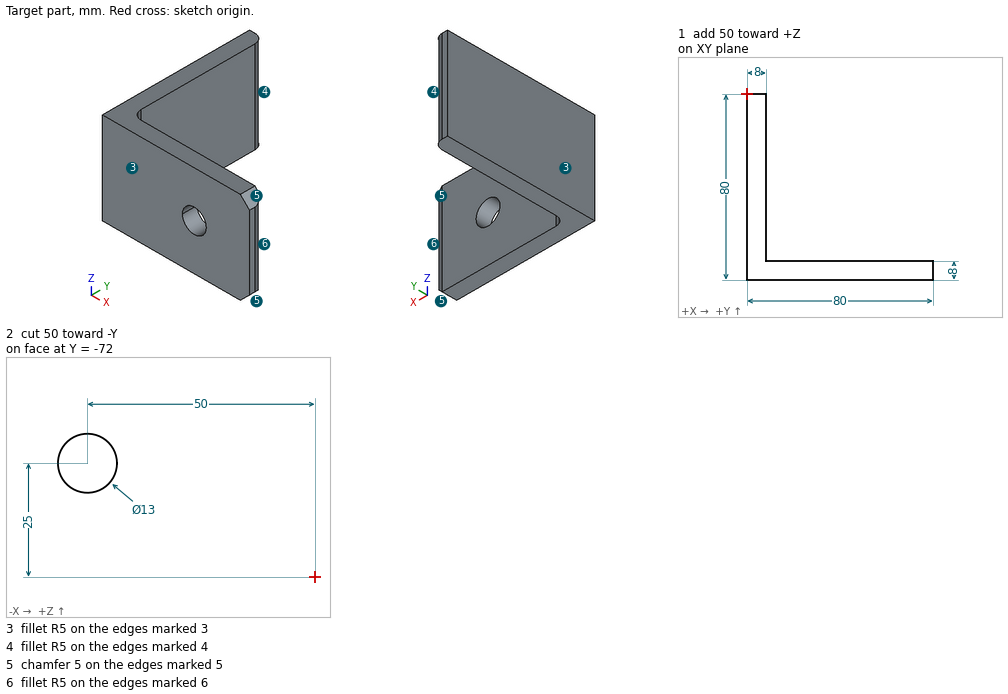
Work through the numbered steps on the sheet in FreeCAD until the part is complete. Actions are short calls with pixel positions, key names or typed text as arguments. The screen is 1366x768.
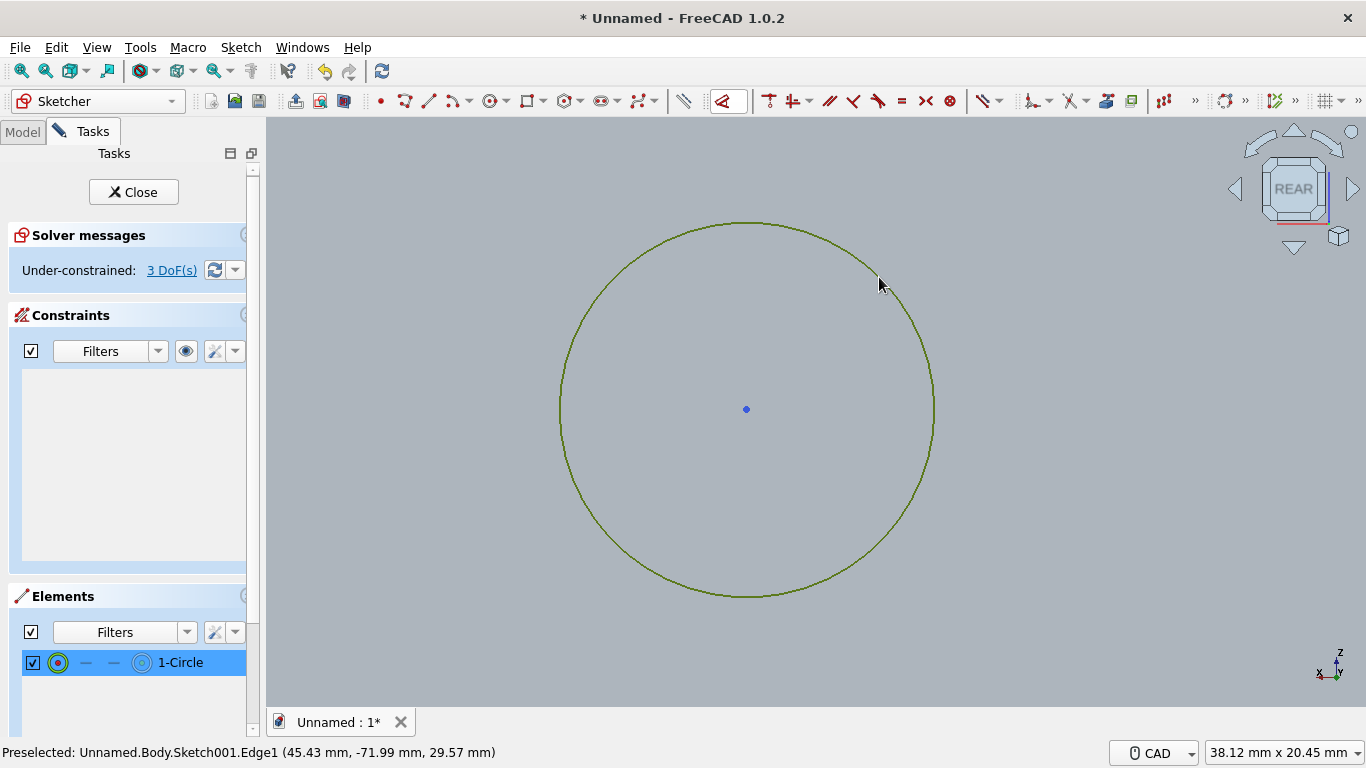
key(k)
key(o)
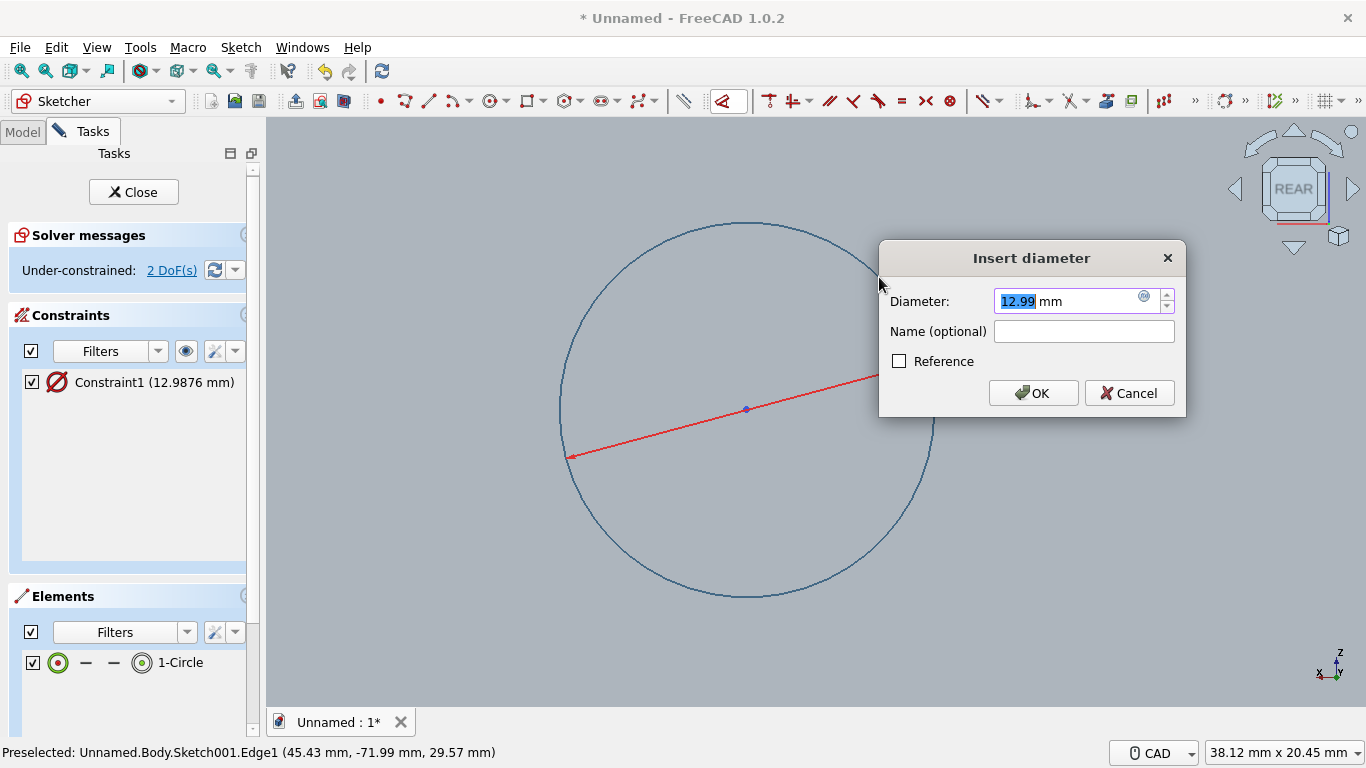
text(13)
key(Return)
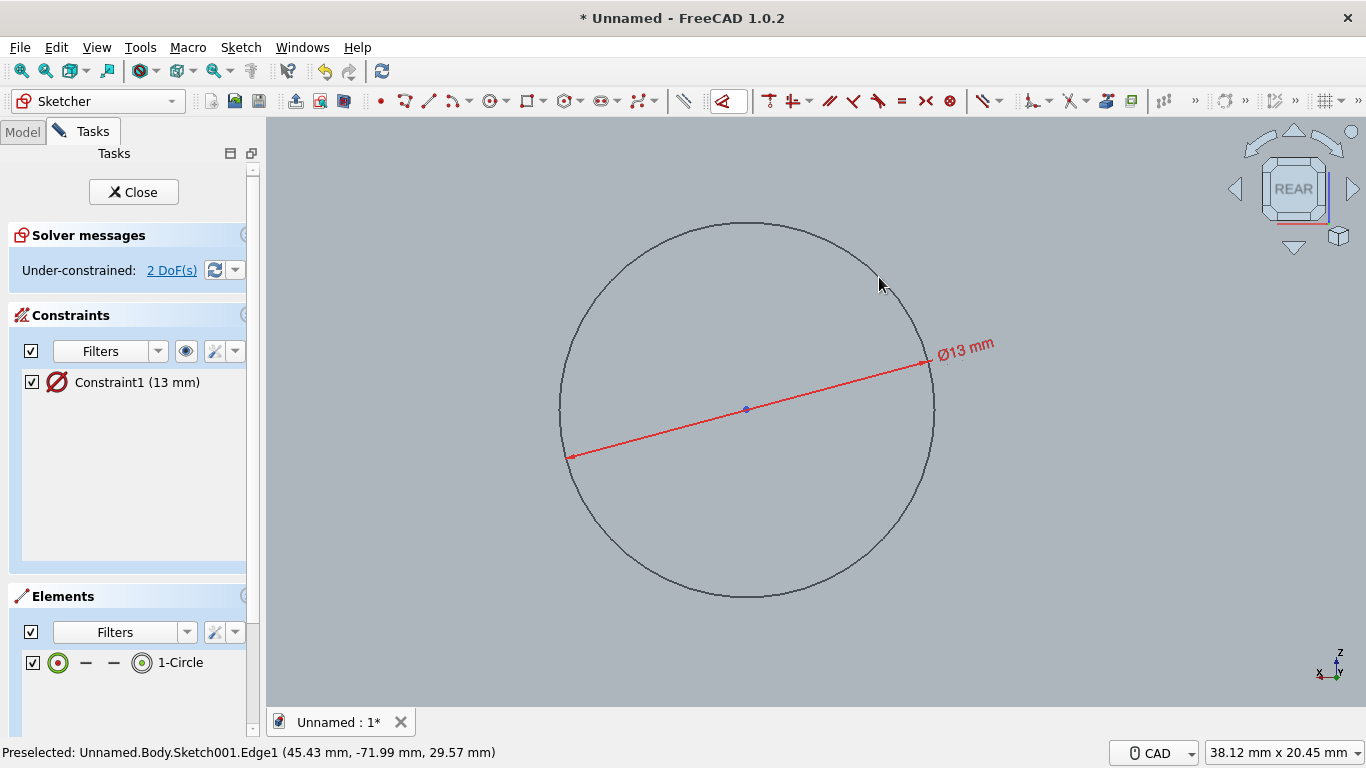
click(747, 410)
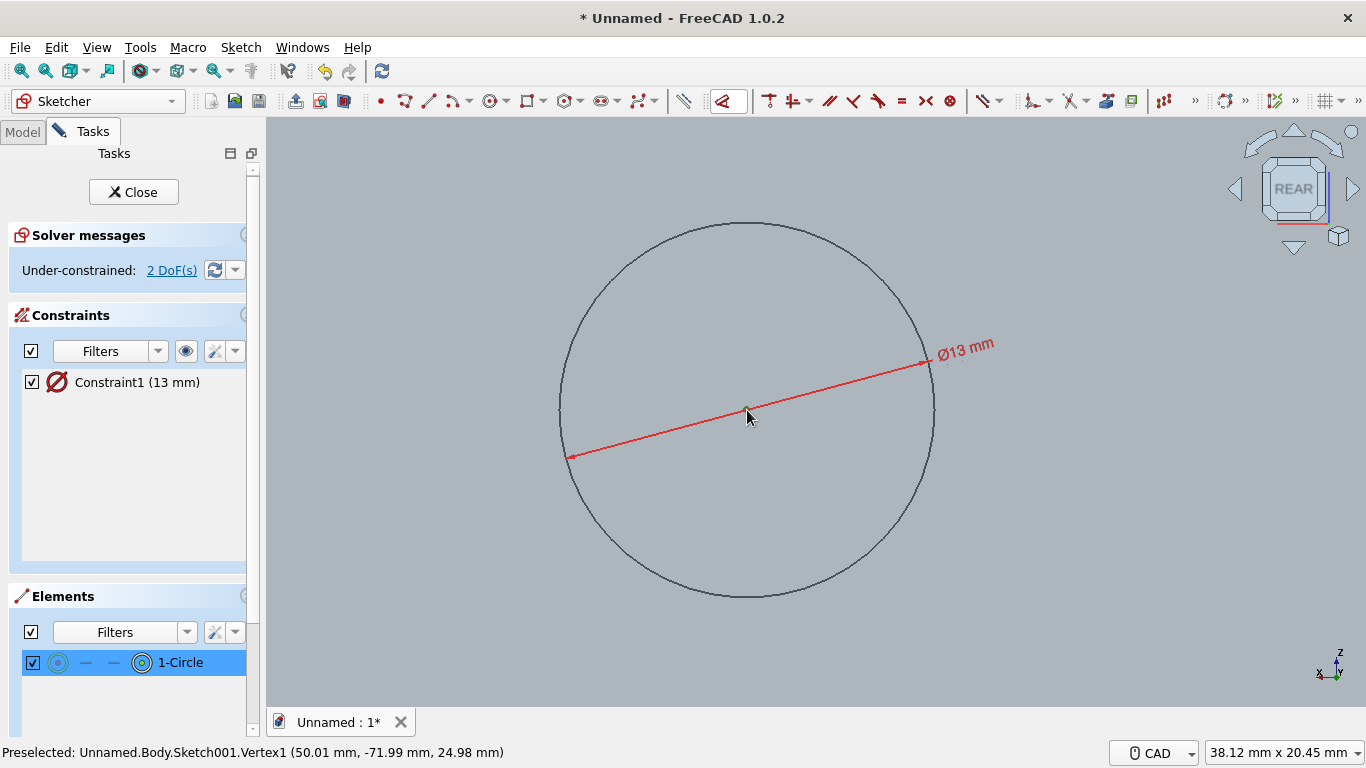
click(742, 102)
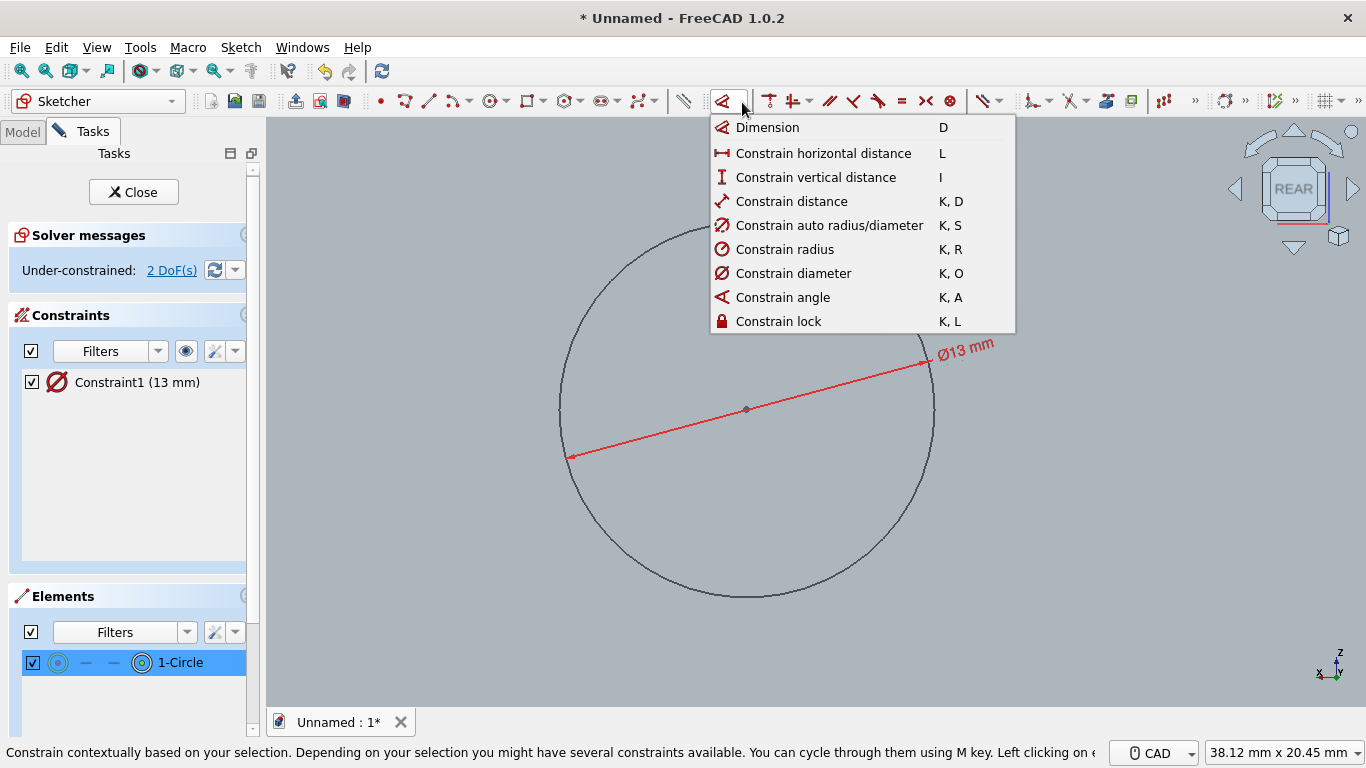
click(863, 153)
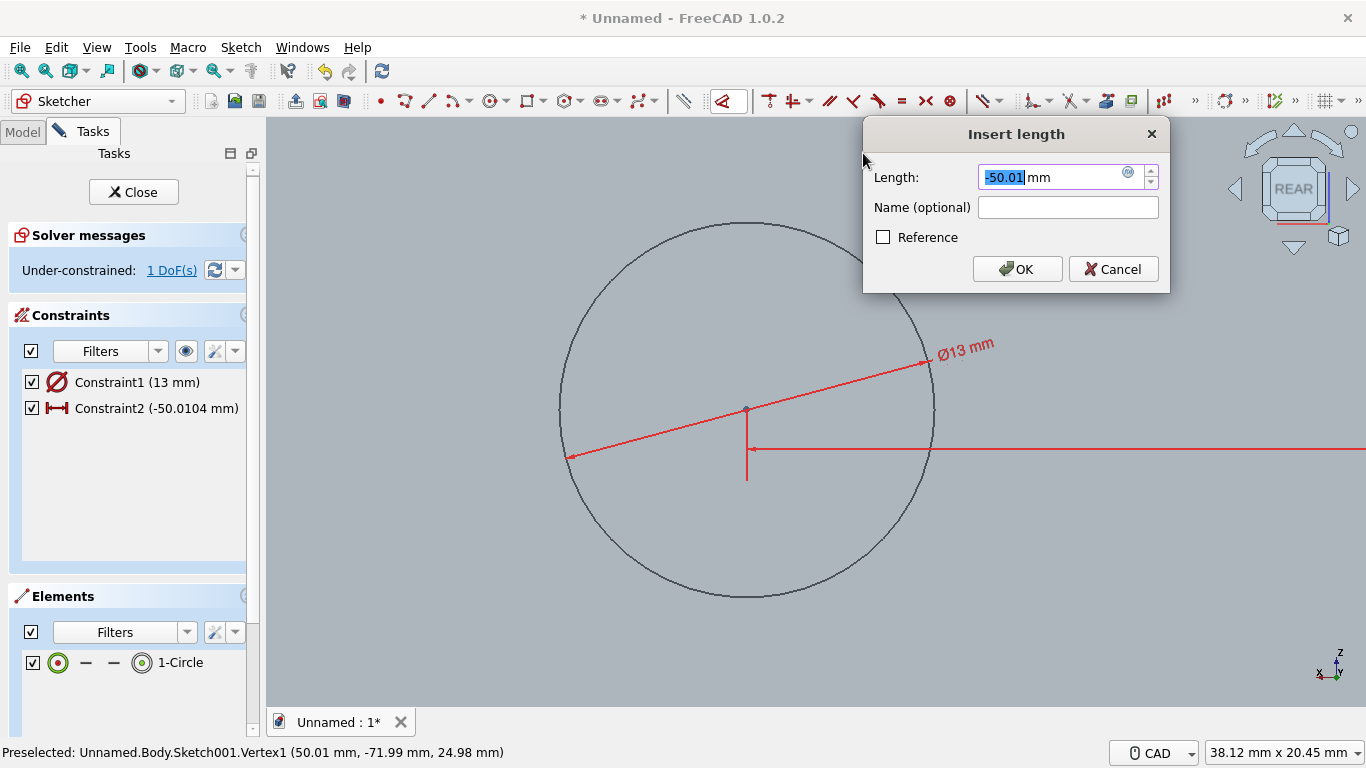
text(-50)
key(Return)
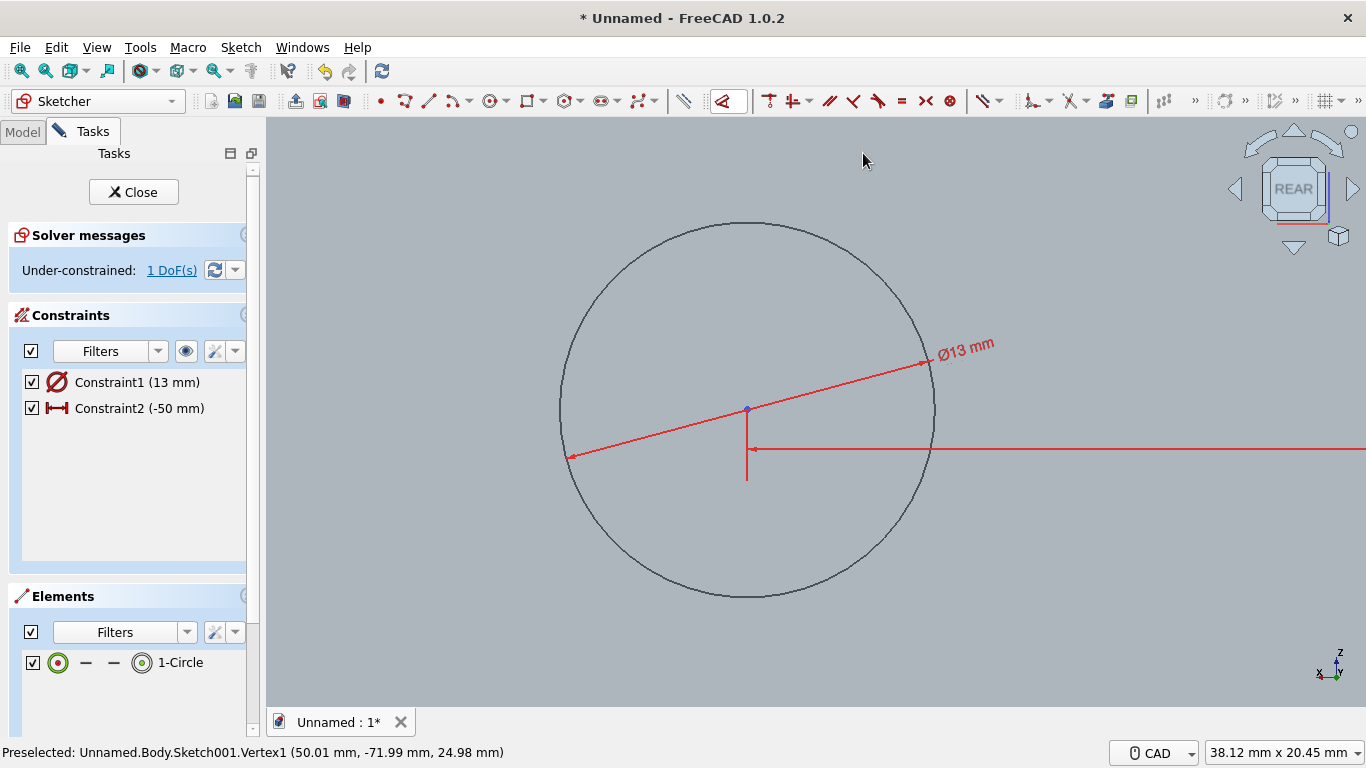
click(747, 410)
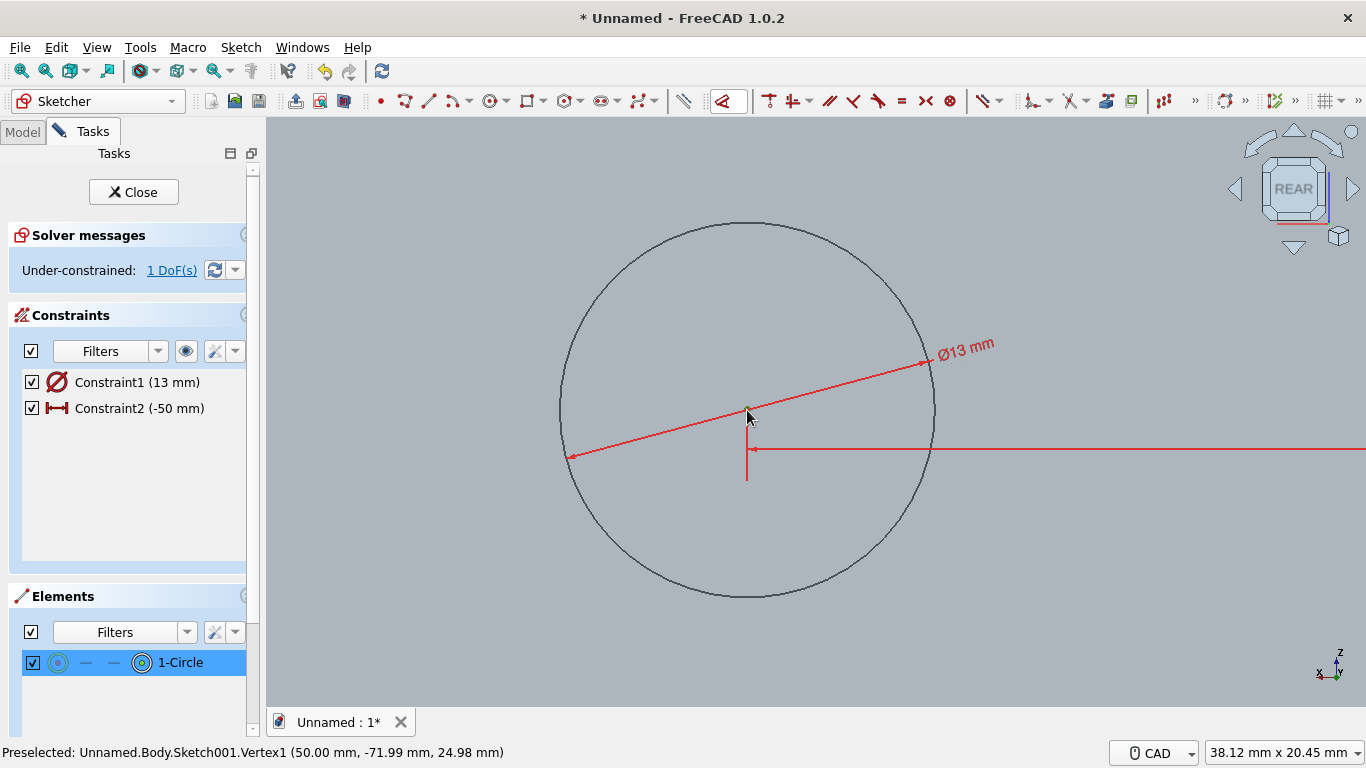
key(i)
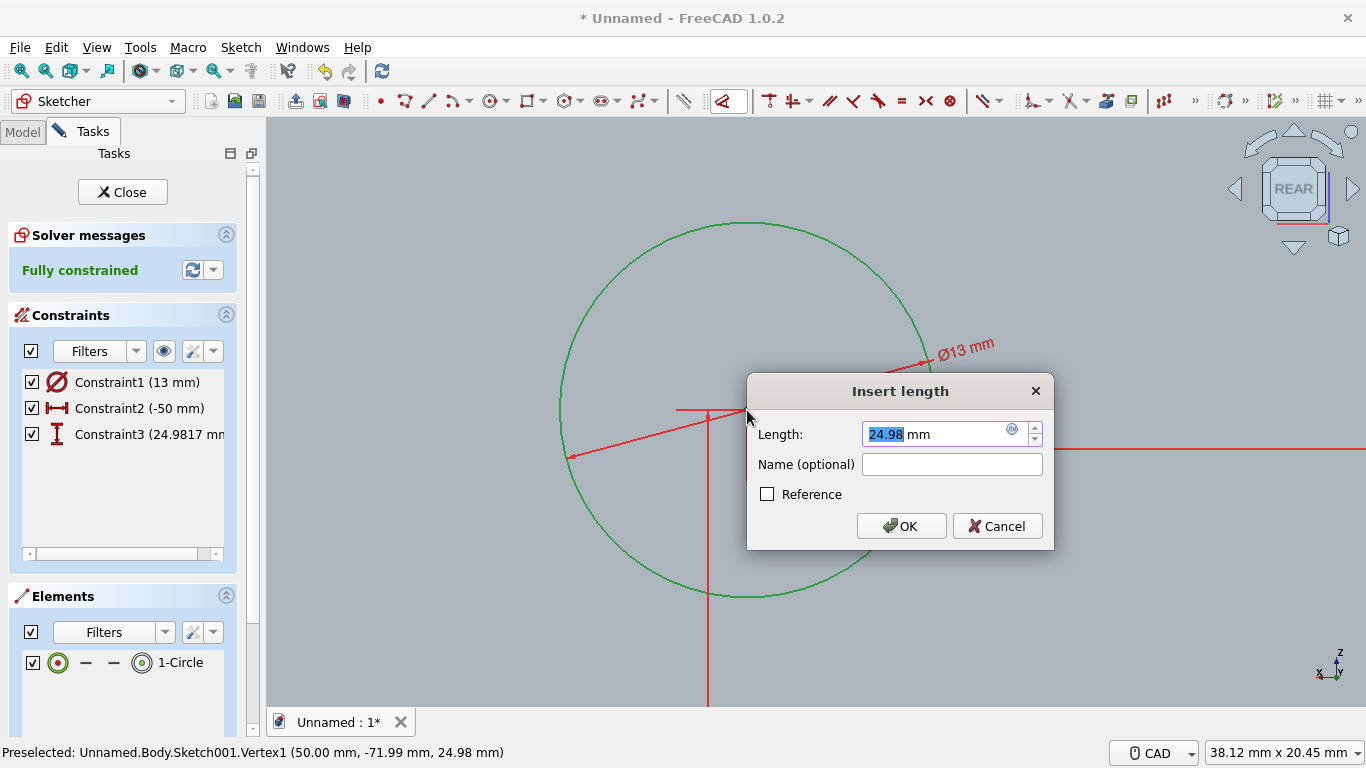
text(25)
key(Return)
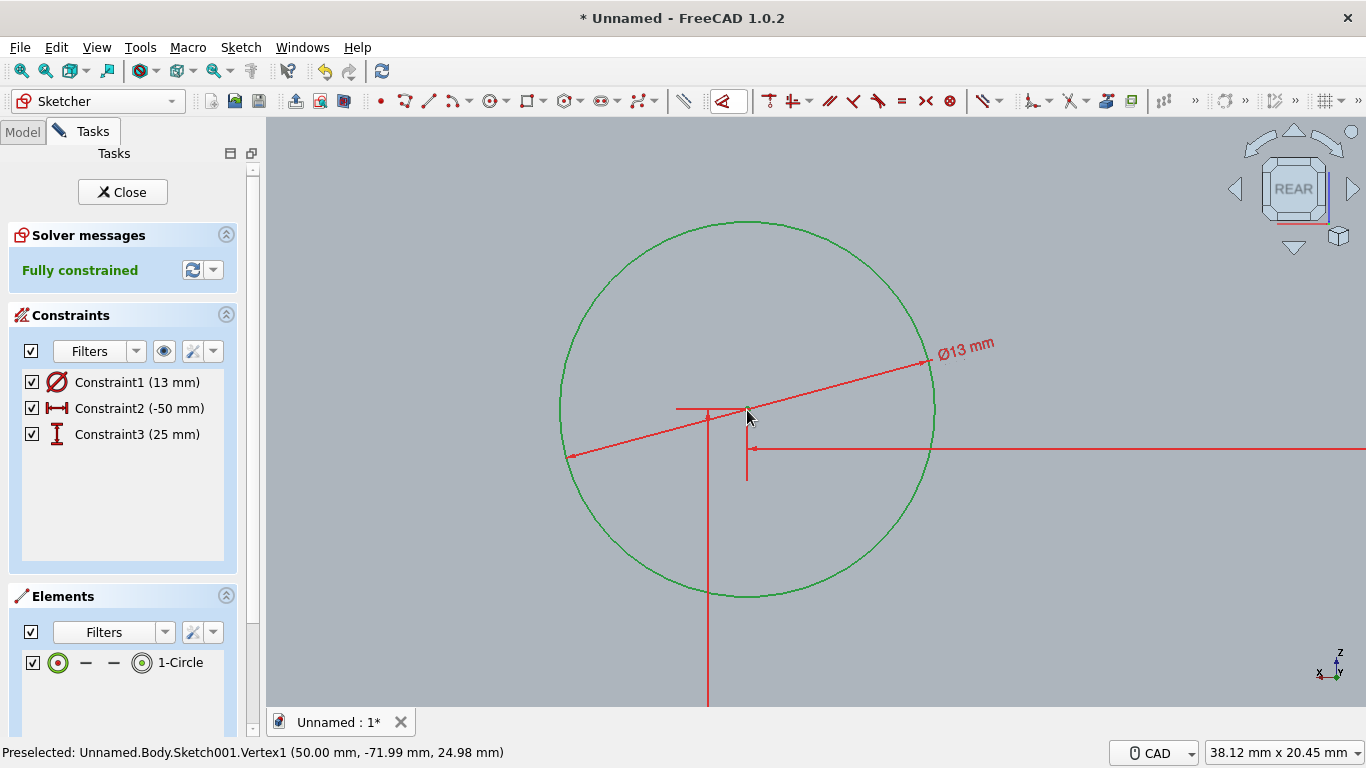
click(123, 192)